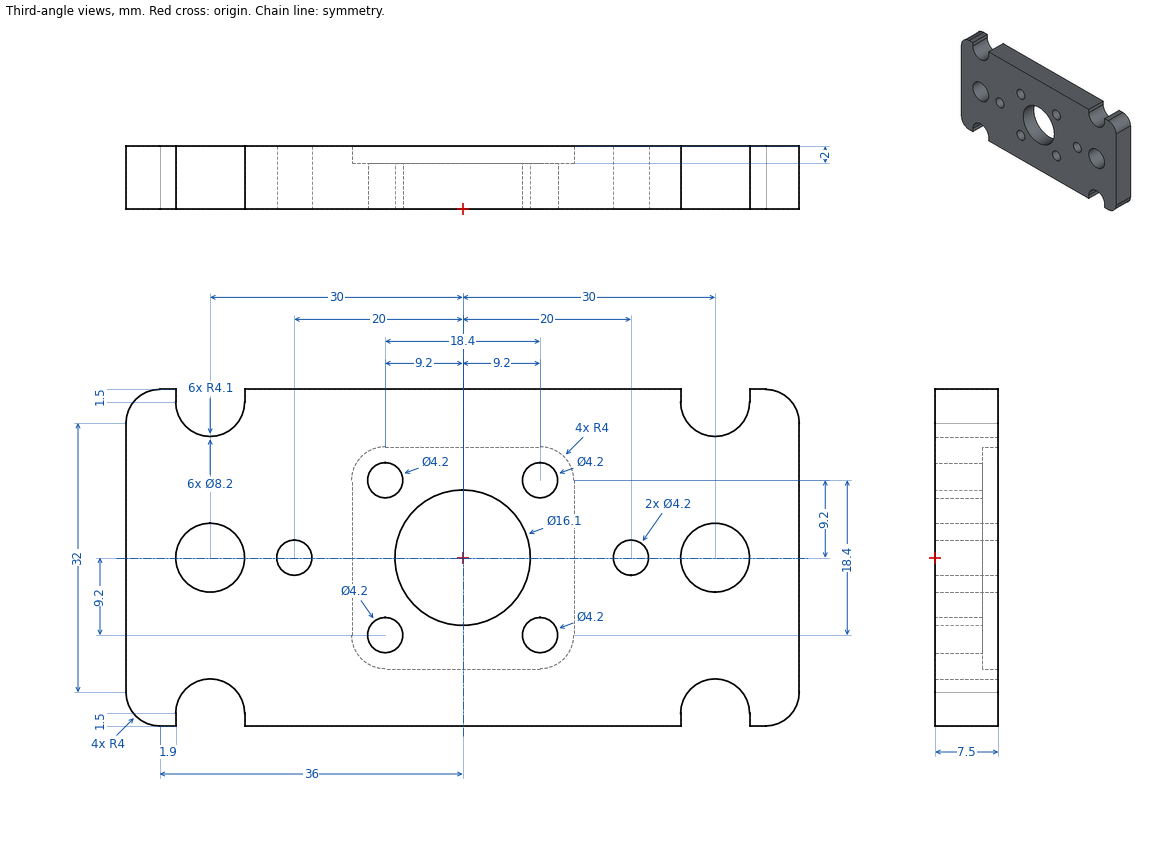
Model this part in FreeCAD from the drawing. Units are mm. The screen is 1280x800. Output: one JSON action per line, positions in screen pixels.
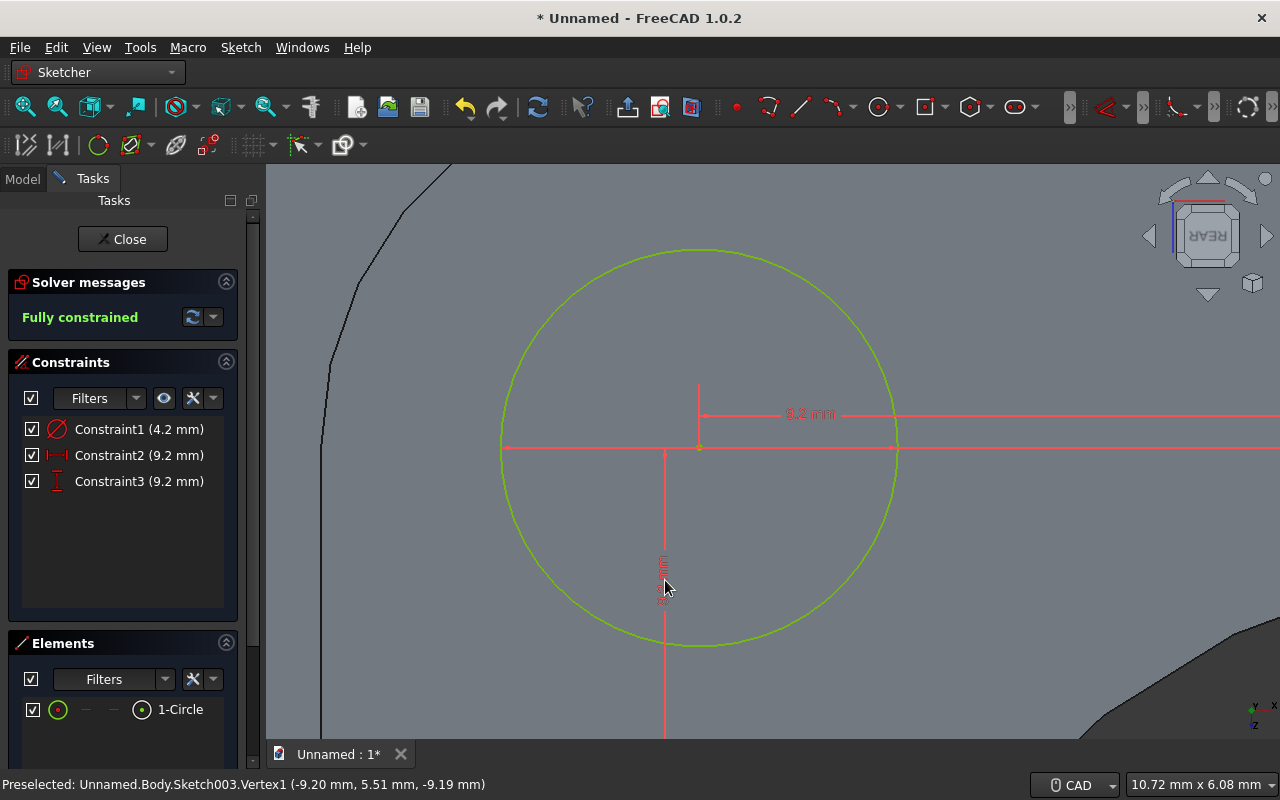
{"action": "left_click", "coordinate": [123, 239]}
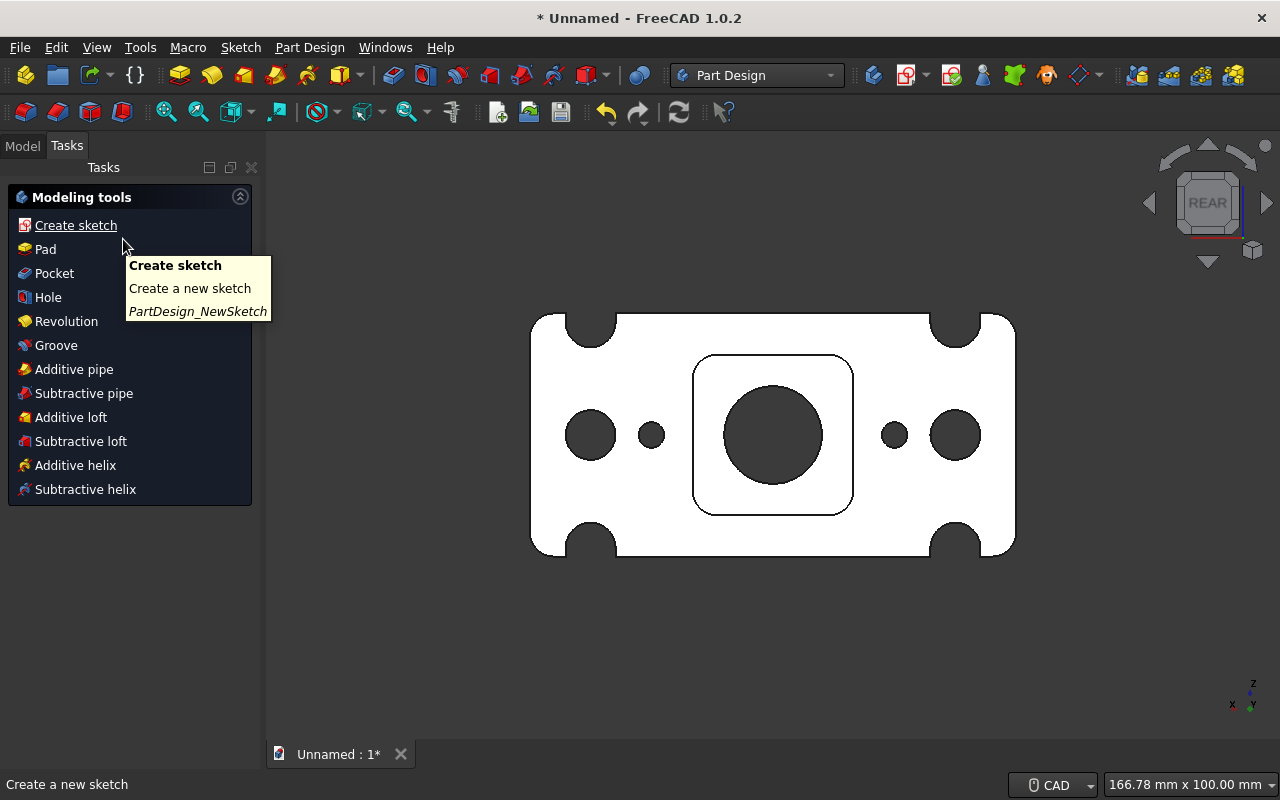
{"action": "left_click", "coordinate": [394, 76]}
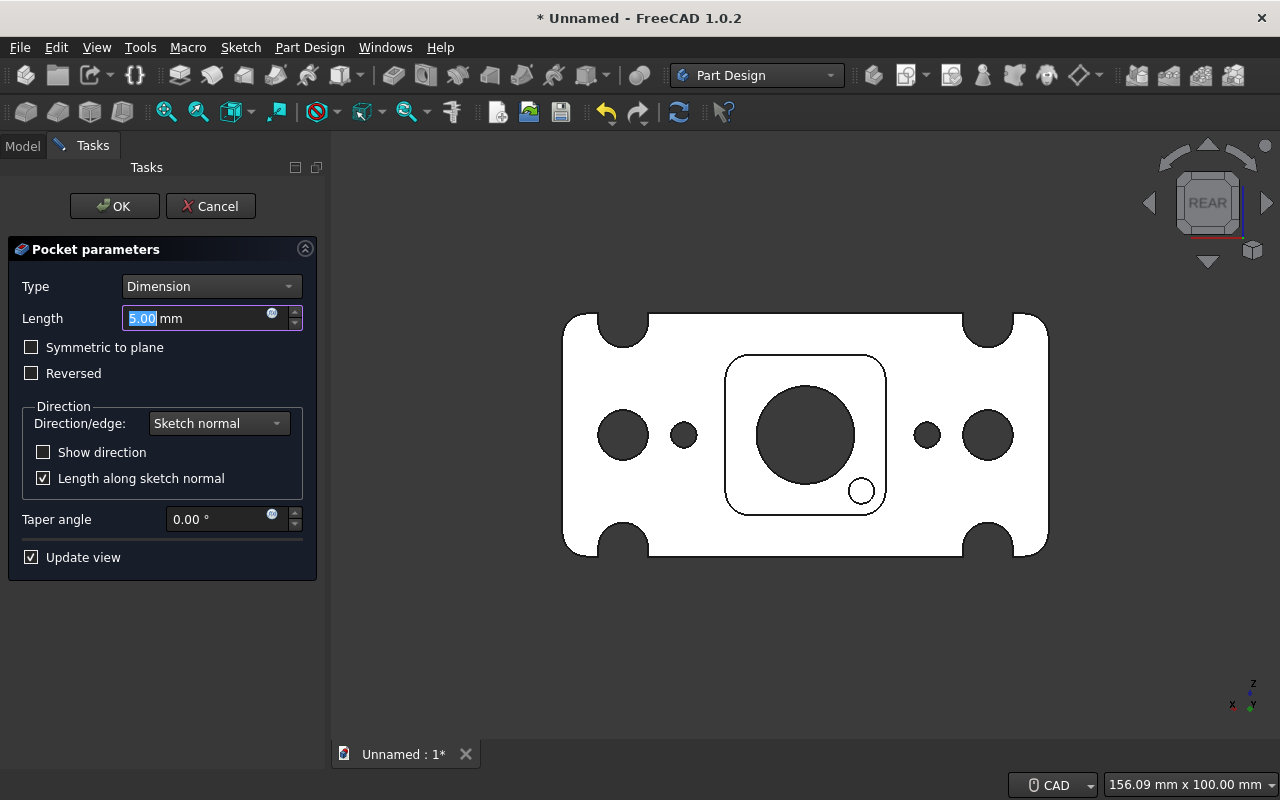
{"action": "left_click", "coordinate": [212, 286]}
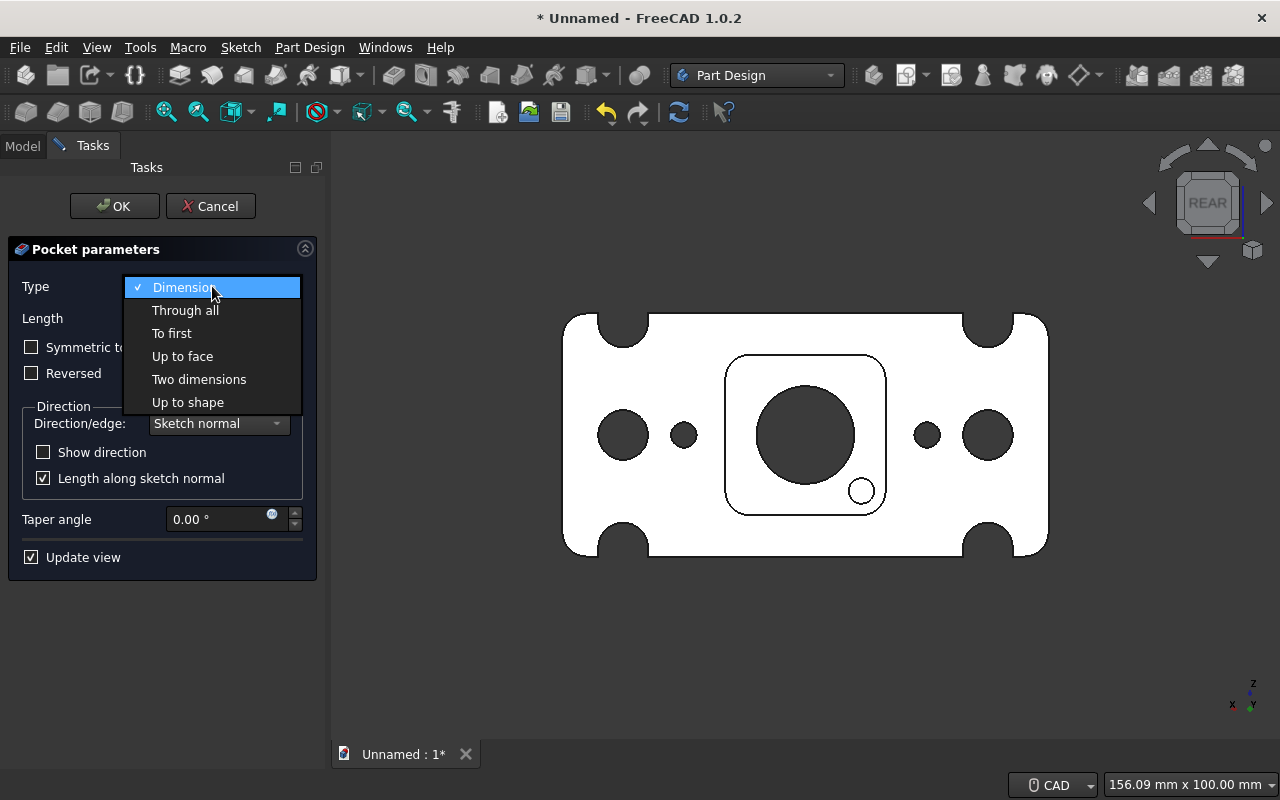
{"action": "left_click", "coordinate": [212, 334]}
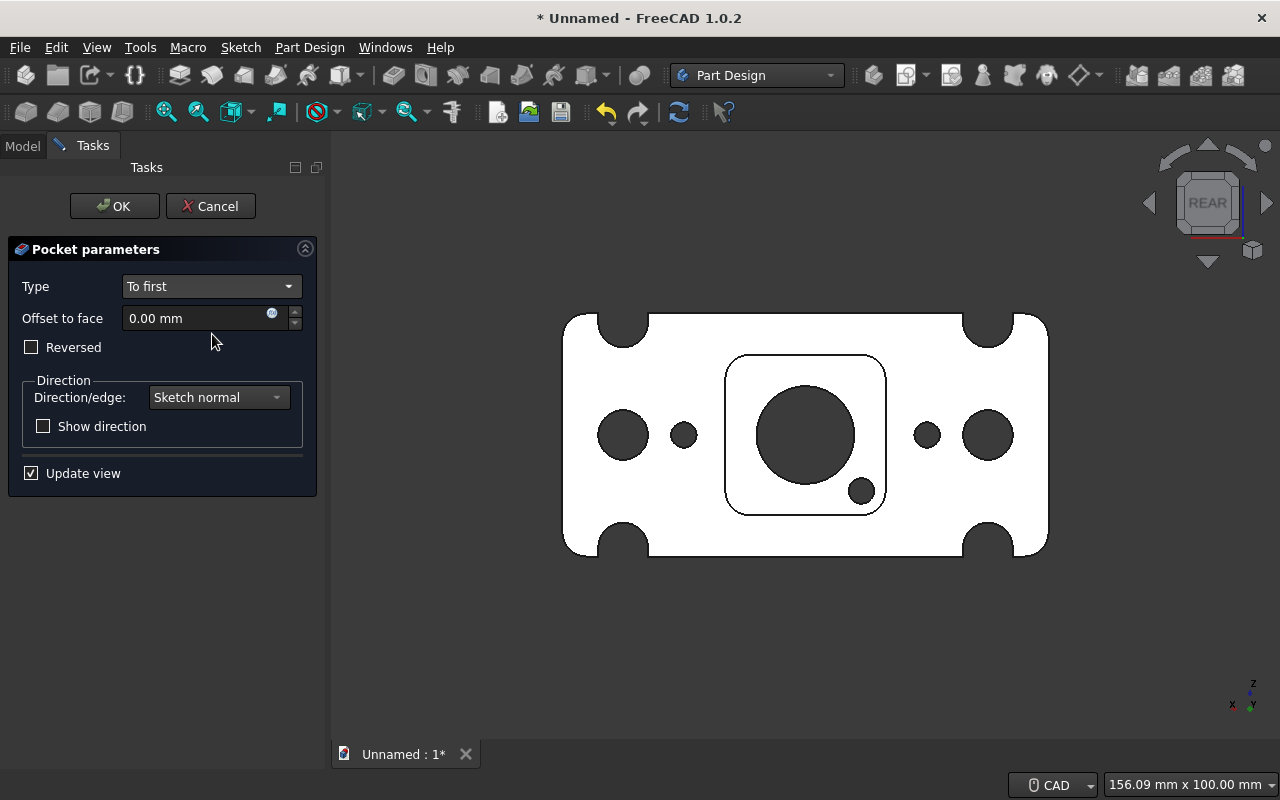
{"action": "left_click", "coordinate": [115, 206]}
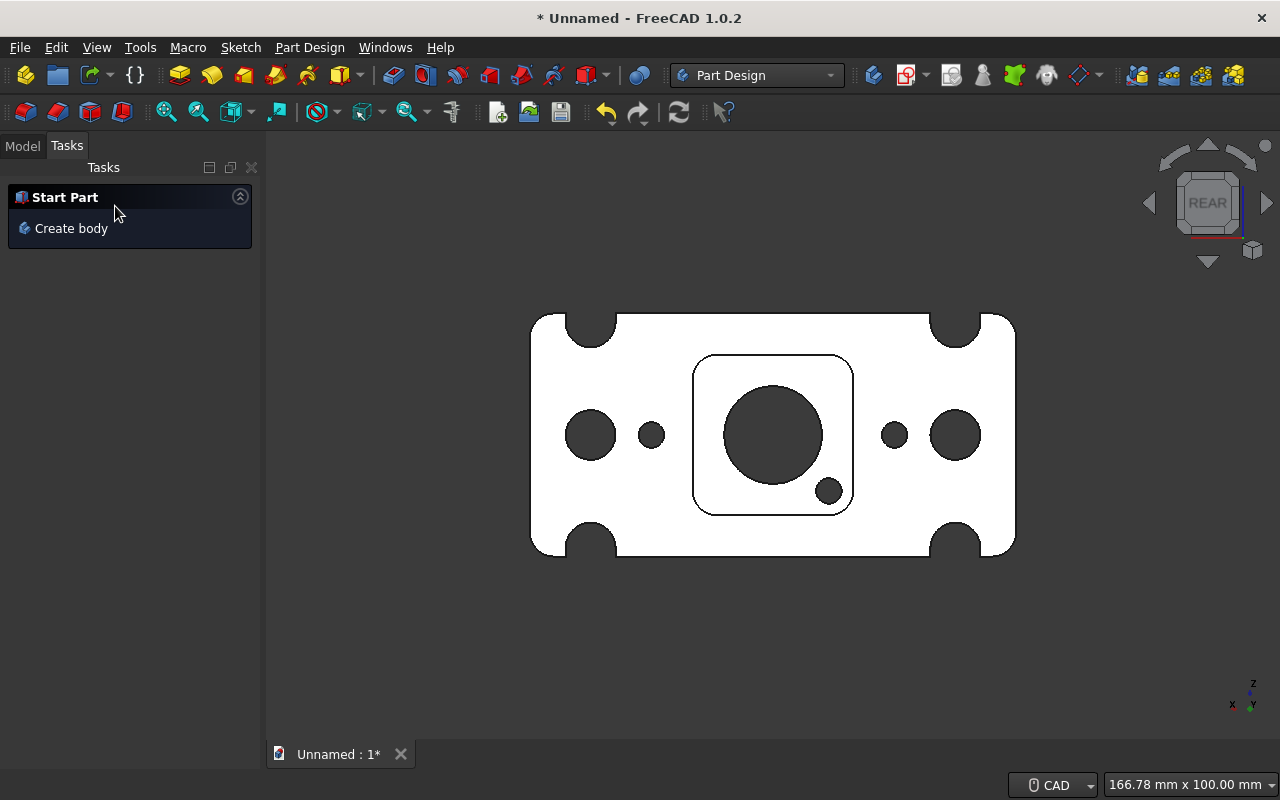
{"action": "left_click", "coordinate": [819, 388]}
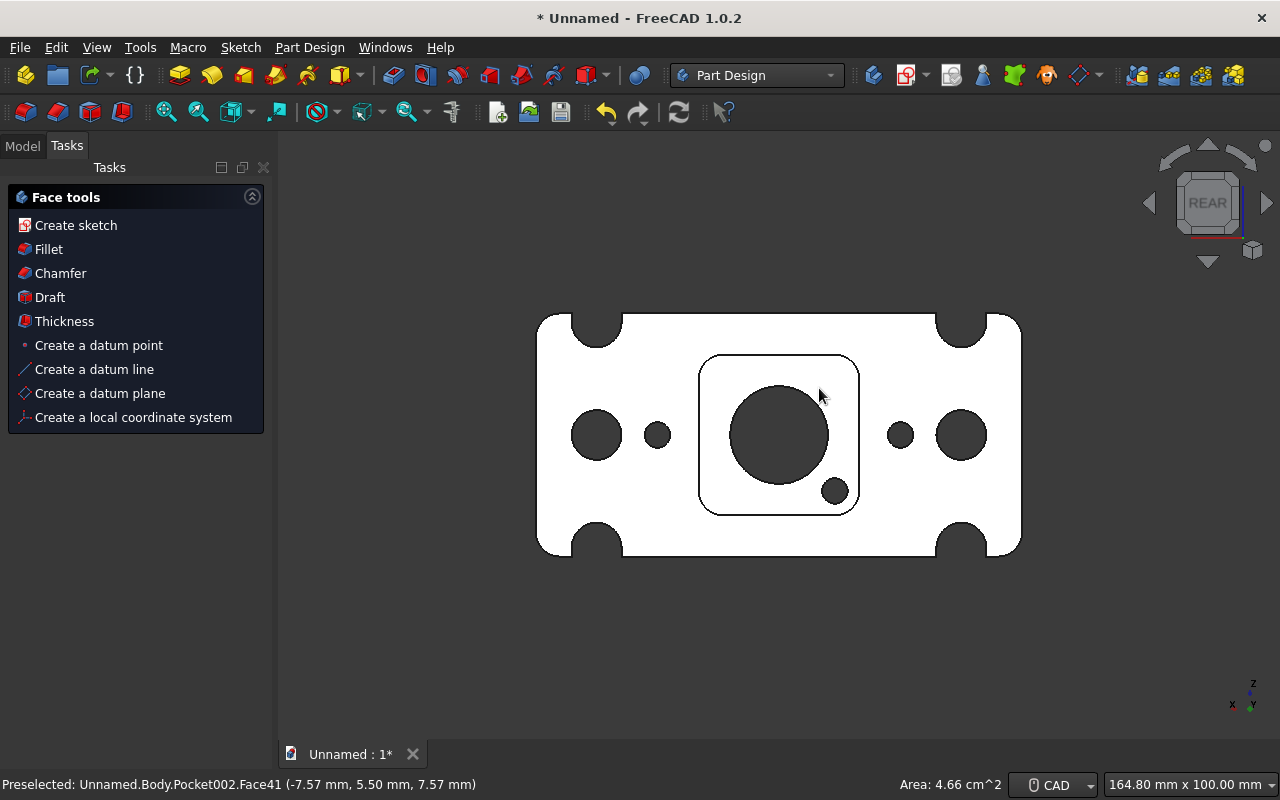
{"action": "left_click", "coordinate": [906, 76]}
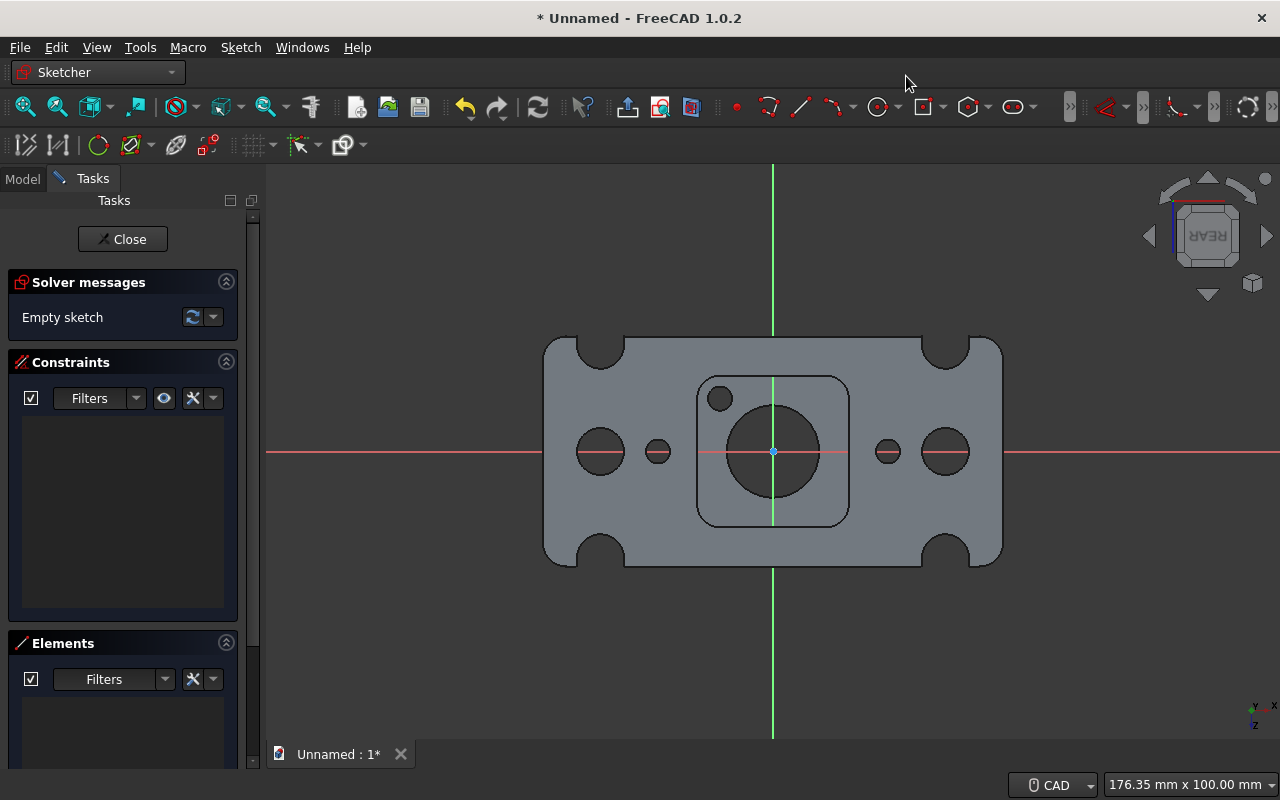
{"action": "scroll", "coordinate": [721, 508], "scroll_direction": "up", "scroll_amount": 14}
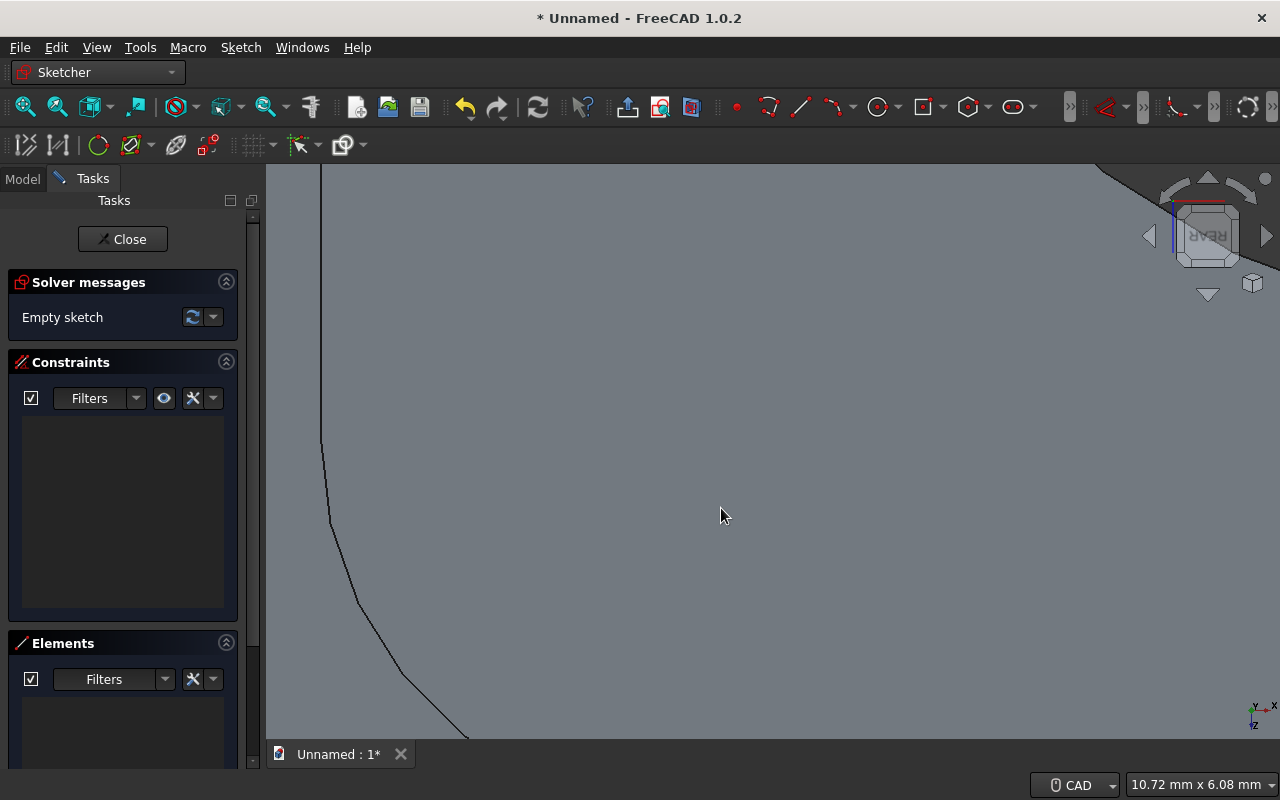
{"action": "left_click", "coordinate": [878, 108]}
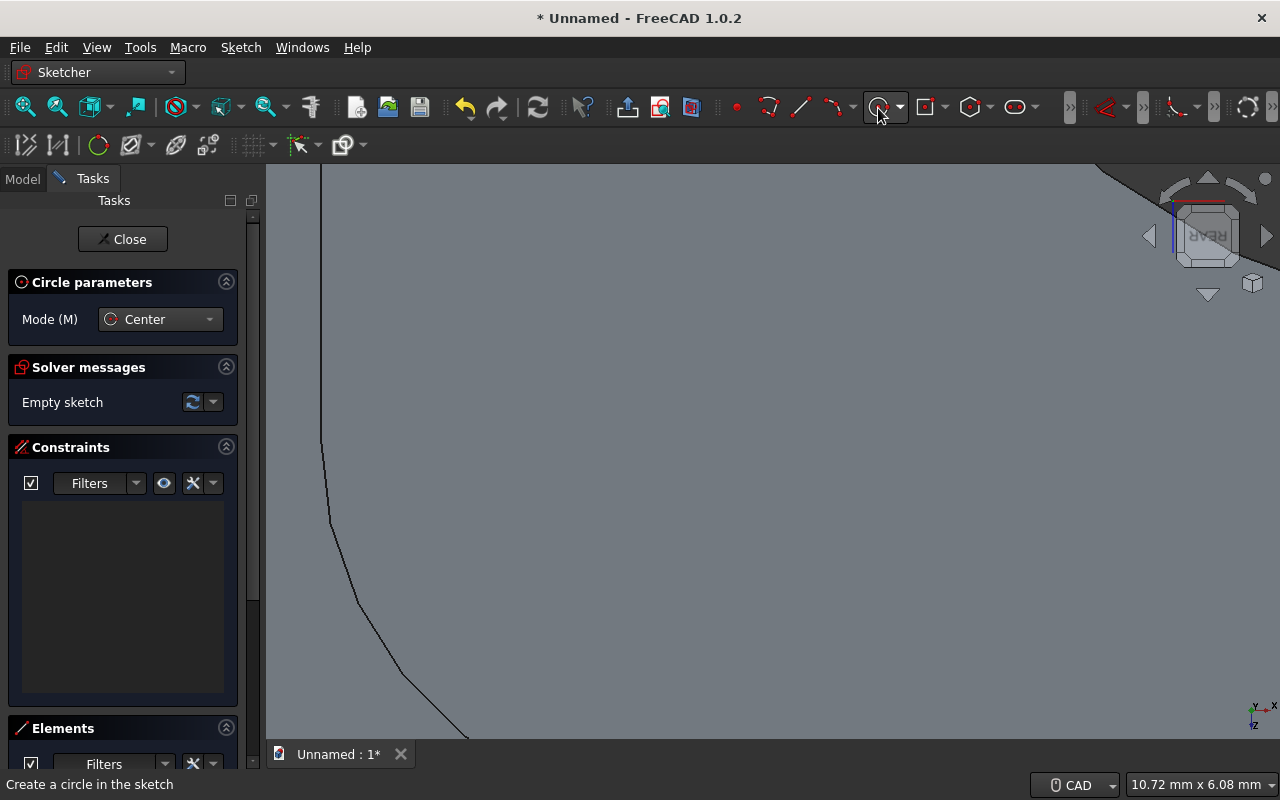
{"action": "left_click", "coordinate": [699, 440]}
{"action": "mouse_move", "coordinate": [840, 299]}